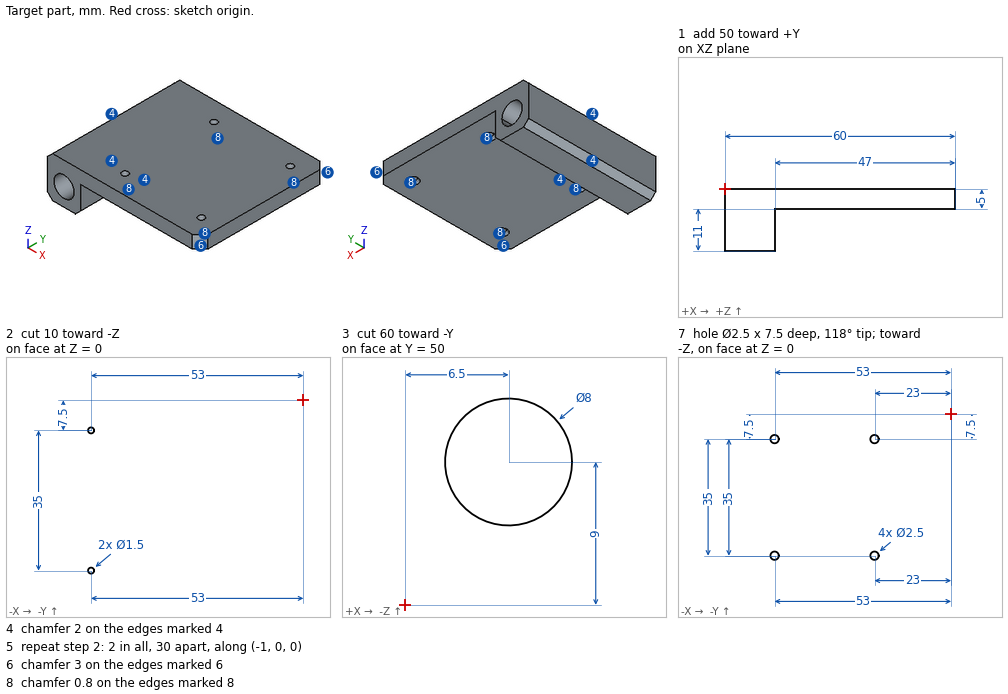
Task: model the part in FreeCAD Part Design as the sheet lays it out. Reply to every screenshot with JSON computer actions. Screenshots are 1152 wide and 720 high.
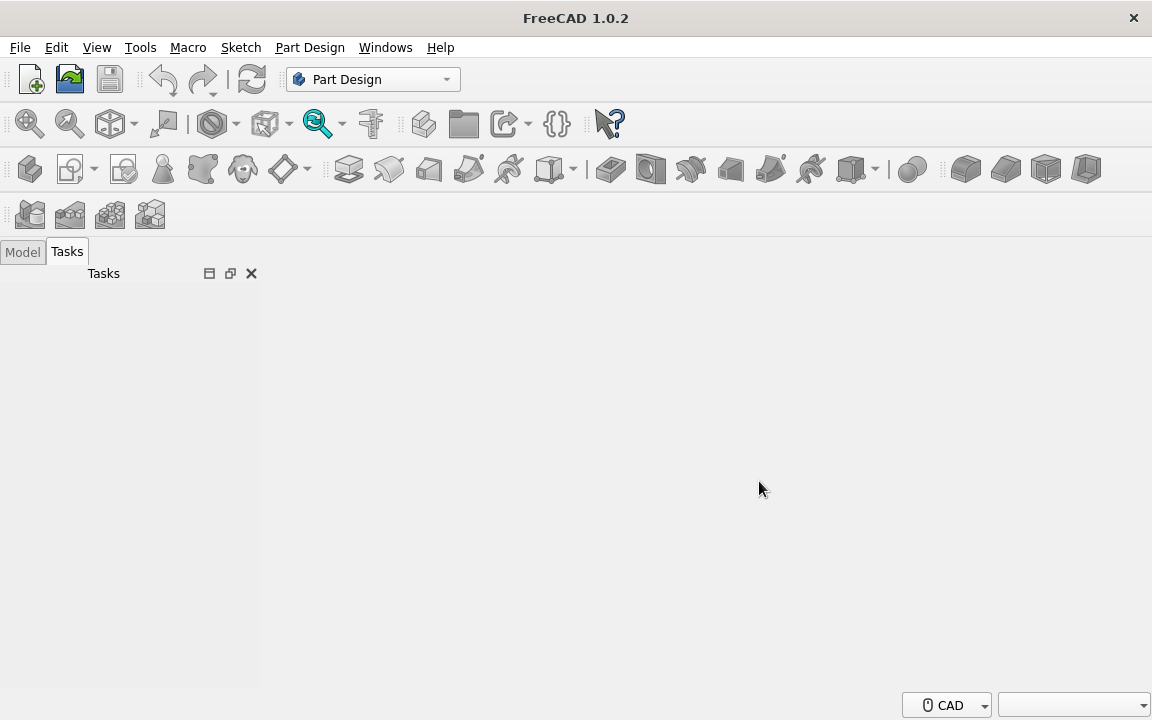
{"action": "left_click", "coordinate": [30, 80]}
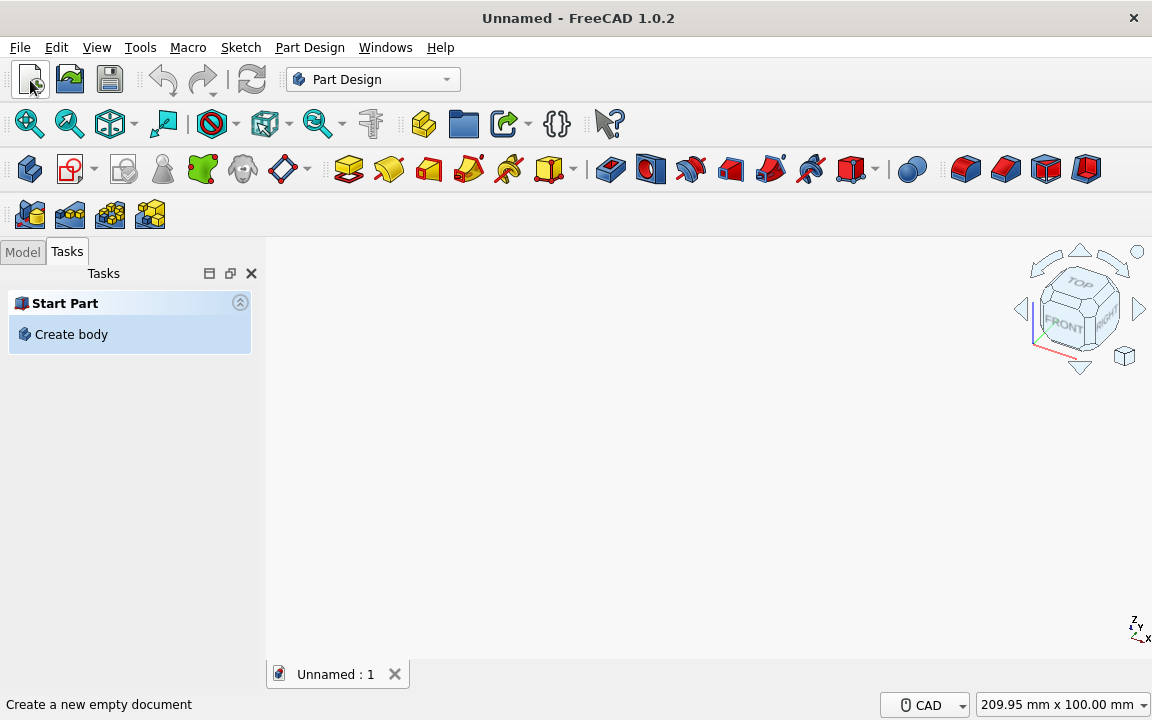
{"action": "left_click", "coordinate": [70, 170]}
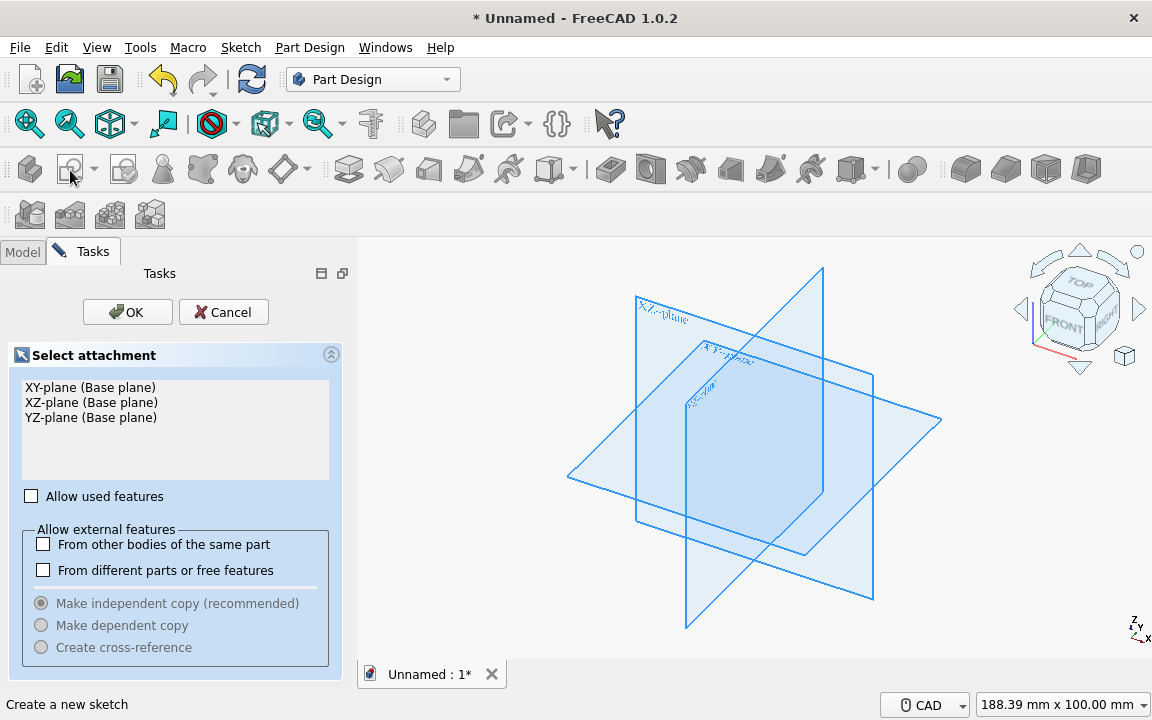
{"action": "left_click", "coordinate": [82, 402]}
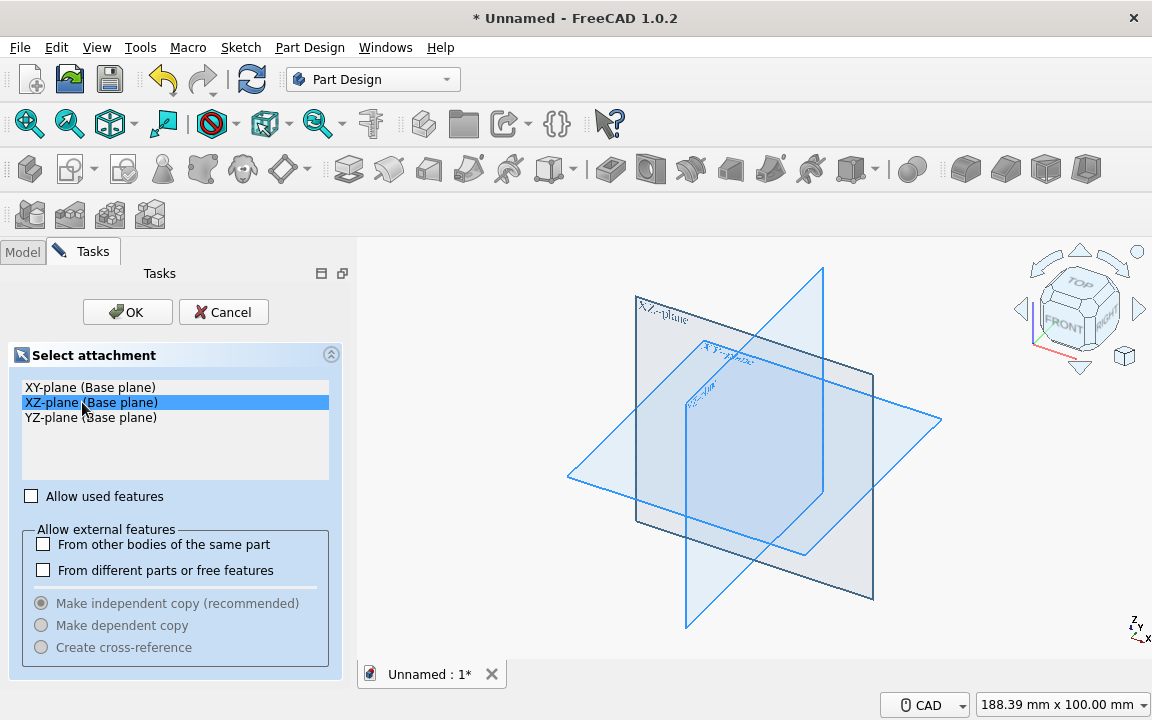
{"action": "left_click", "coordinate": [128, 312]}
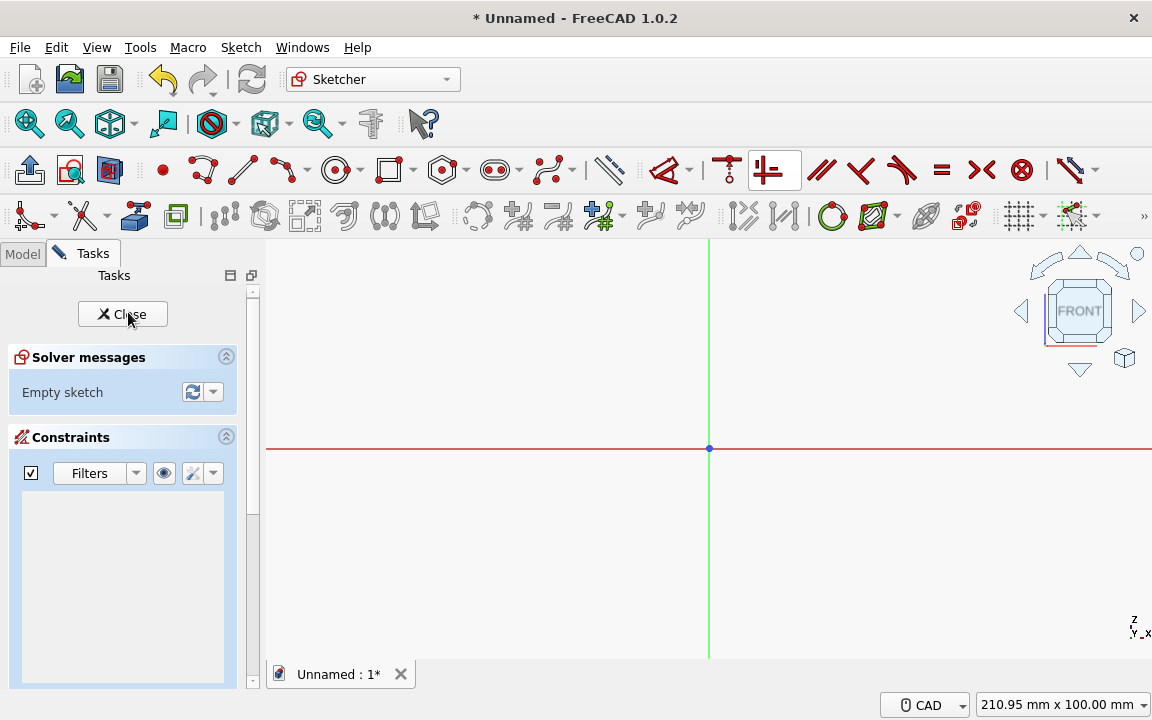
{"action": "scroll", "coordinate": [987, 523], "scroll_direction": "up", "scroll_amount": 3}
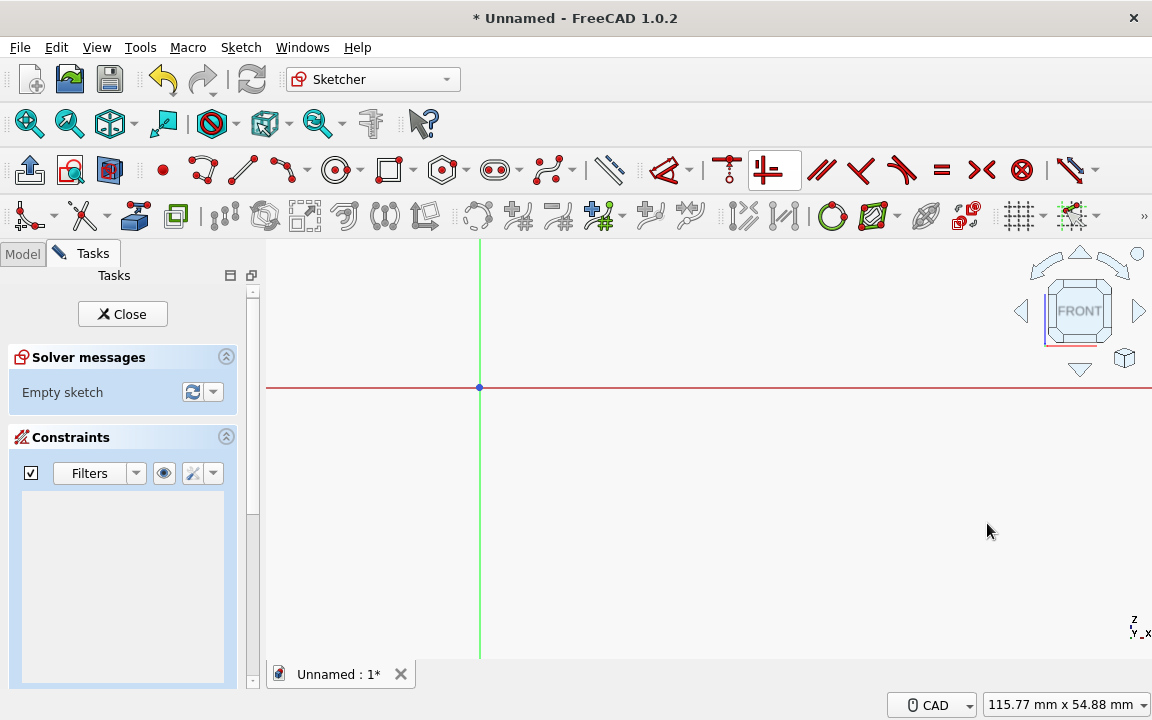
{"action": "left_click", "coordinate": [204, 170]}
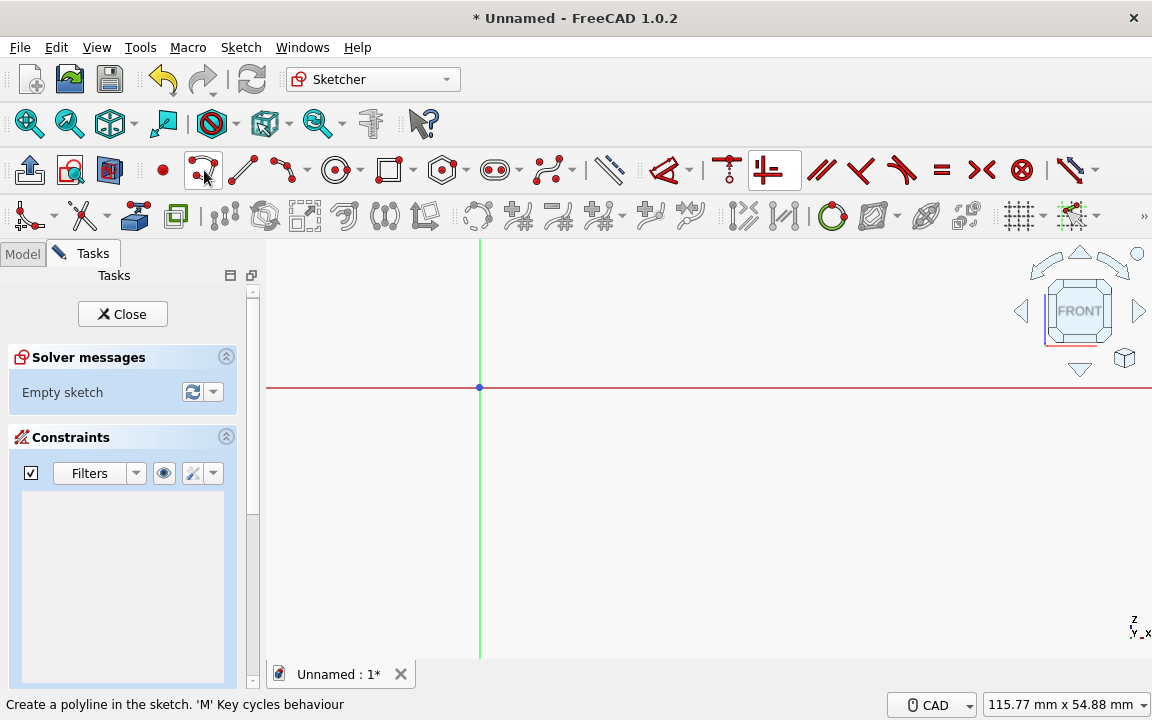
{"action": "left_click", "coordinate": [480, 388]}
{"action": "left_click", "coordinate": [939, 397]}
{"action": "left_click", "coordinate": [939, 426]}
{"action": "left_click", "coordinate": [579, 426]}
{"action": "left_click", "coordinate": [579, 510]}
{"action": "left_click", "coordinate": [489, 510]}
{"action": "left_click", "coordinate": [480, 388]}
{"action": "key", "text": "Escape"}
{"action": "key", "text": "Escape"}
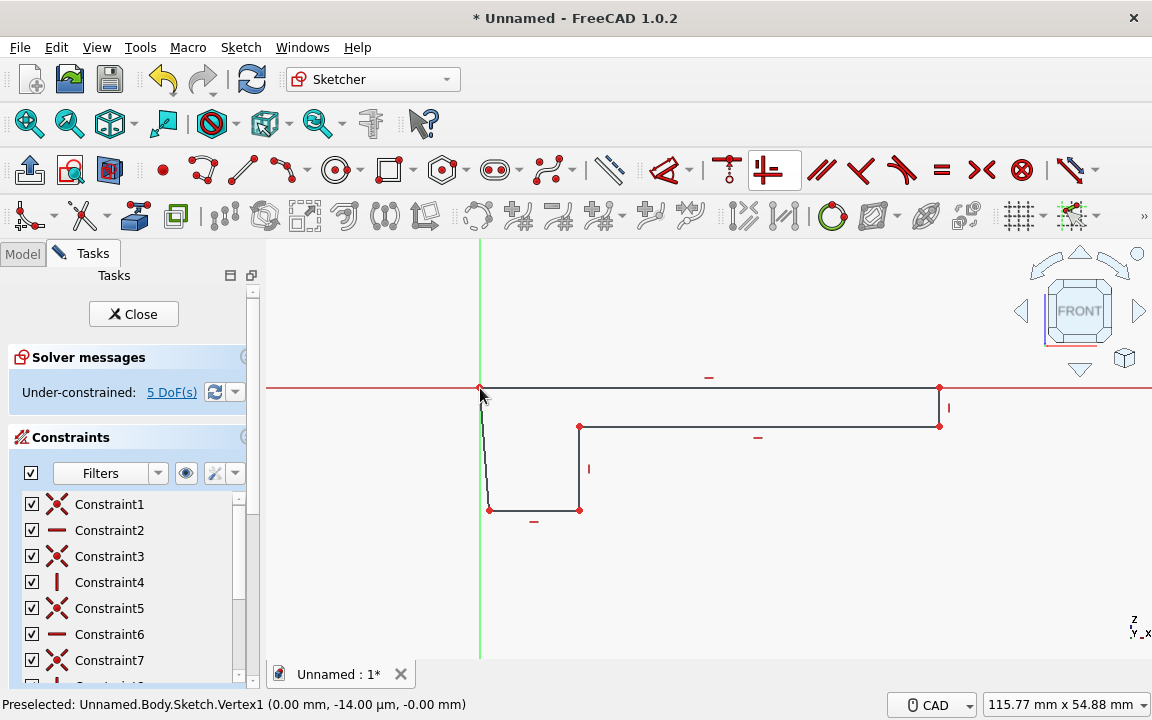
{"action": "left_click", "coordinate": [483, 425]}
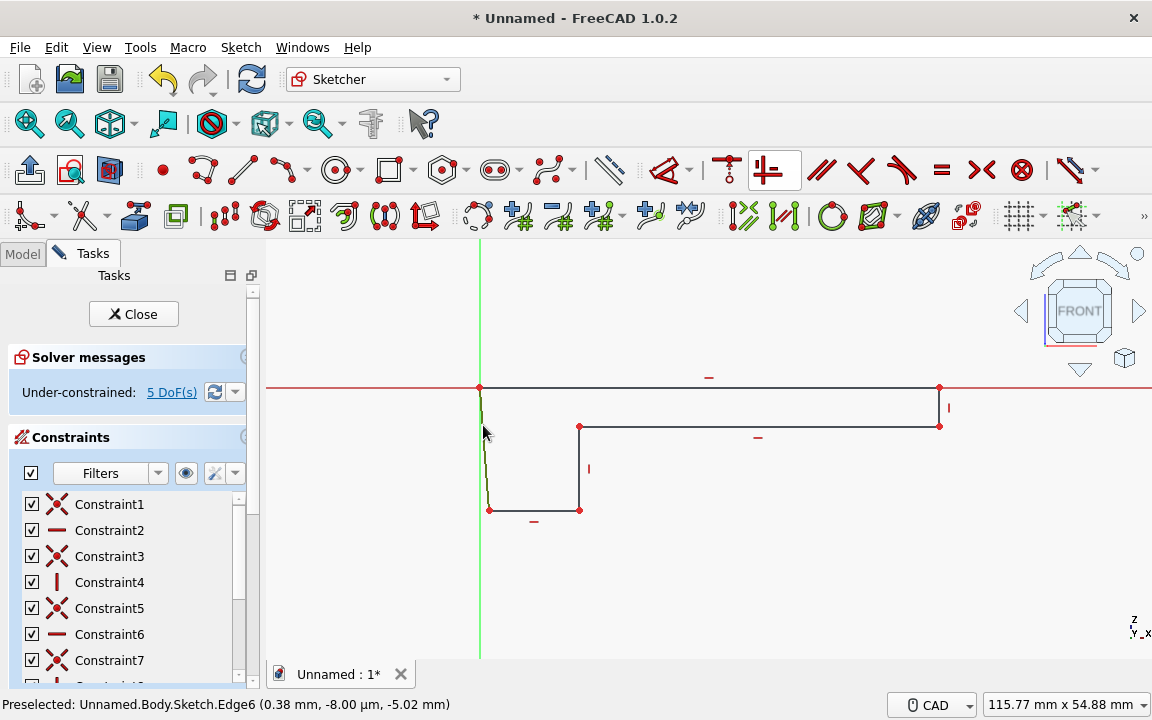
{"action": "key", "text": "v"}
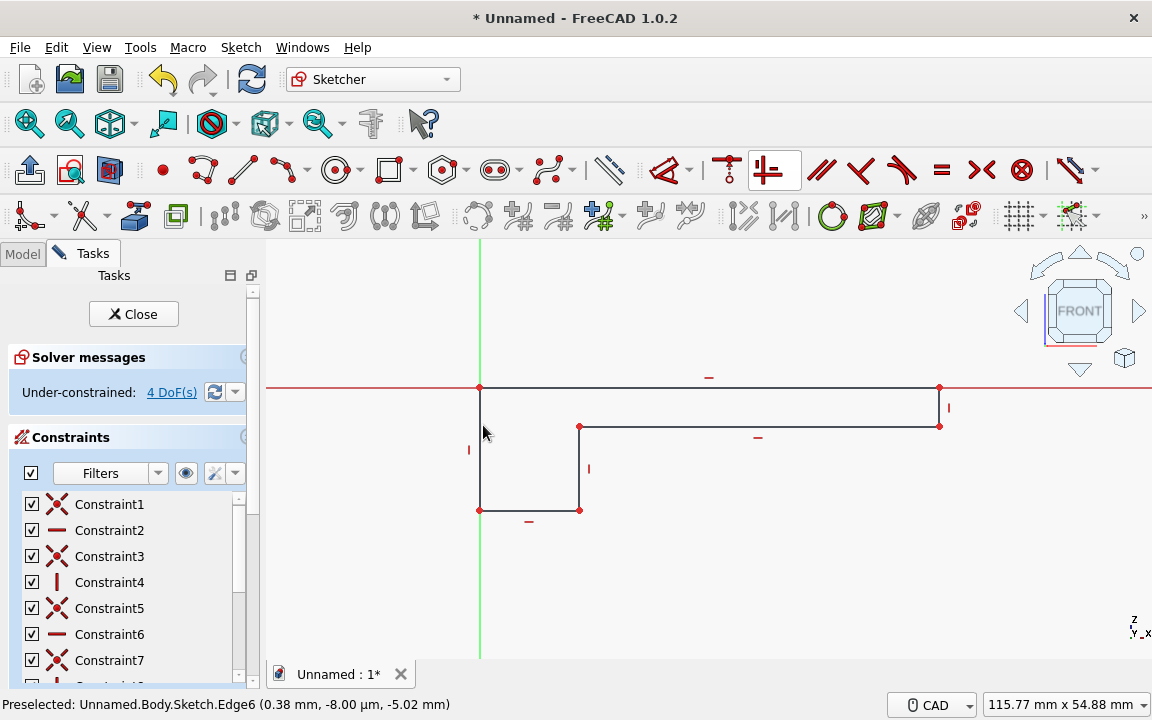
{"action": "left_click", "coordinate": [664, 170]}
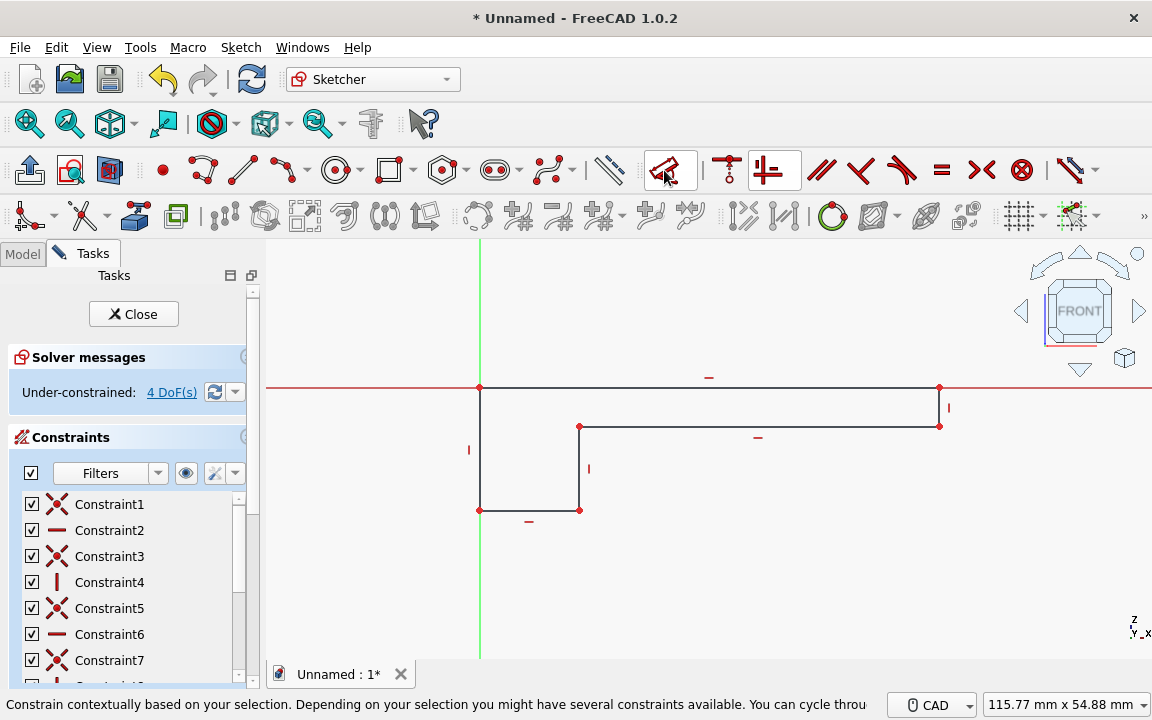
{"action": "left_click", "coordinate": [939, 399]}
{"action": "left_click", "coordinate": [973, 407]}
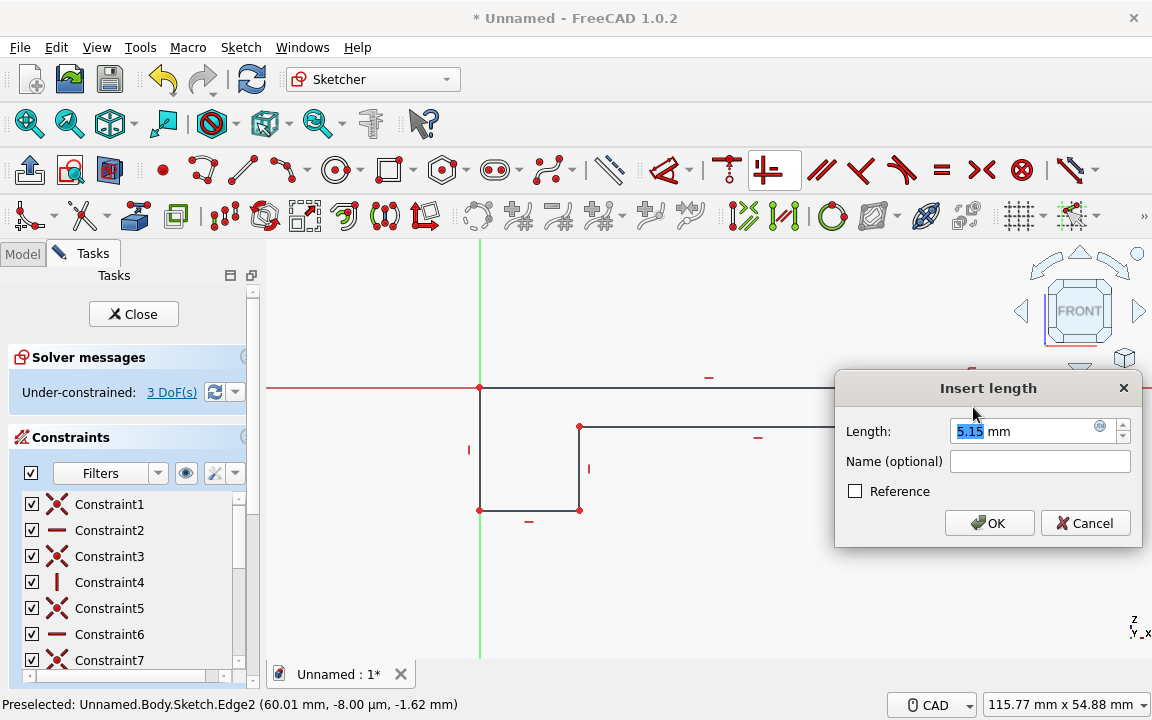
{"action": "type", "text": "5"}
{"action": "key", "text": "Return"}